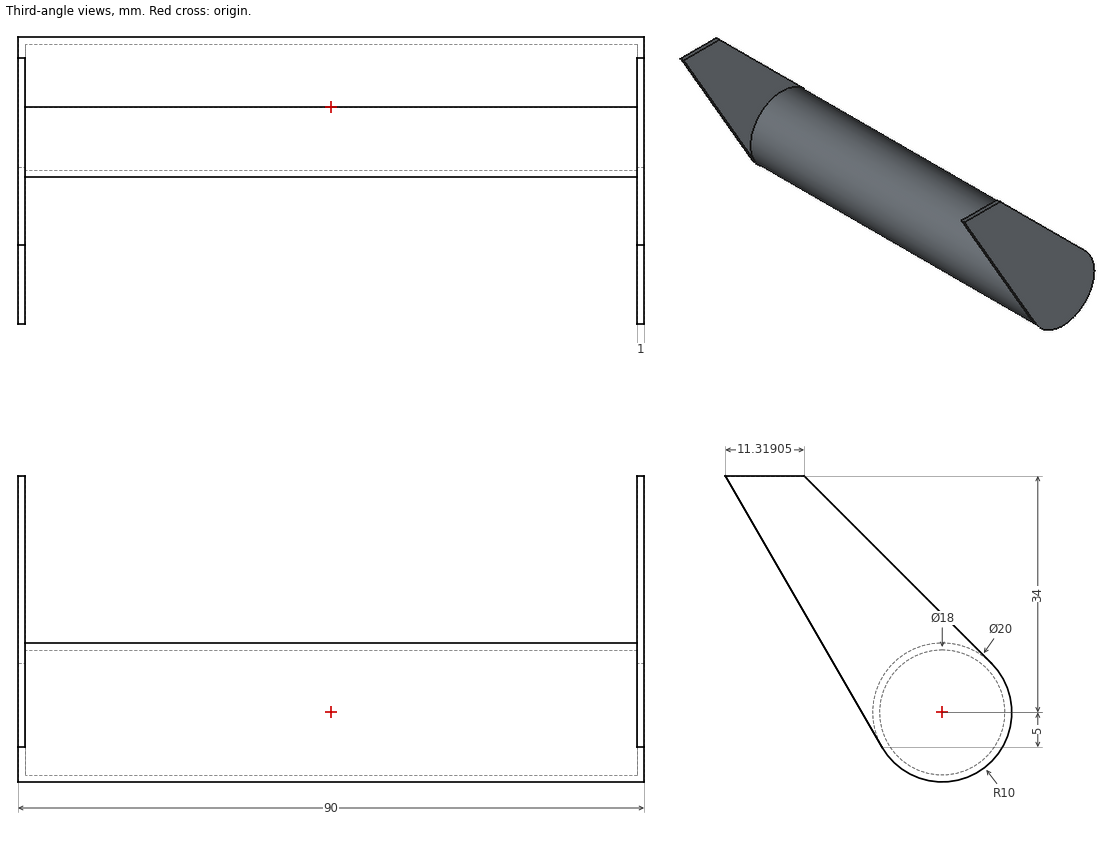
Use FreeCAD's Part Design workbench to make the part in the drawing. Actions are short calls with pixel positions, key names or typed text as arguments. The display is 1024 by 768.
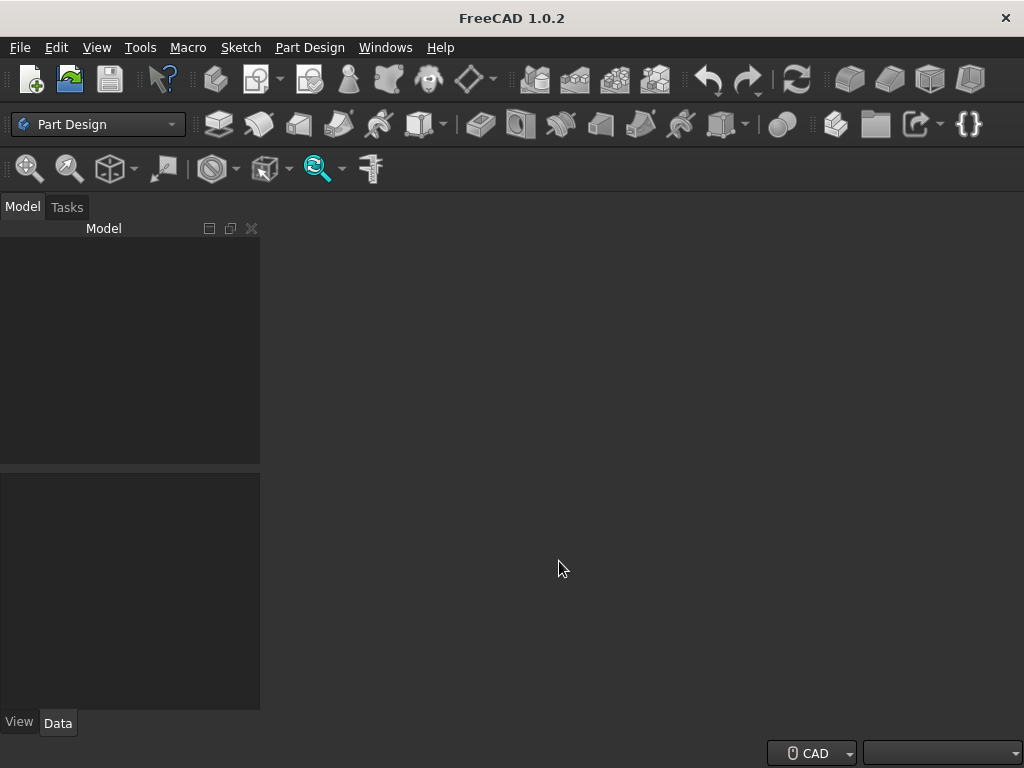
click(30, 80)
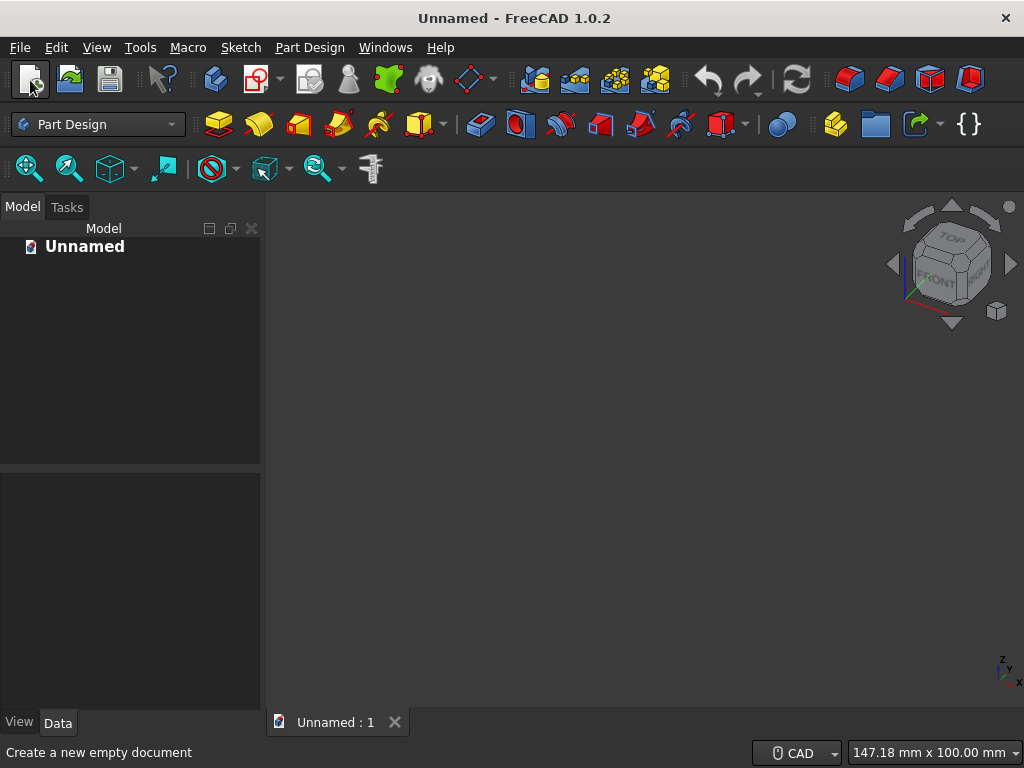
click(256, 80)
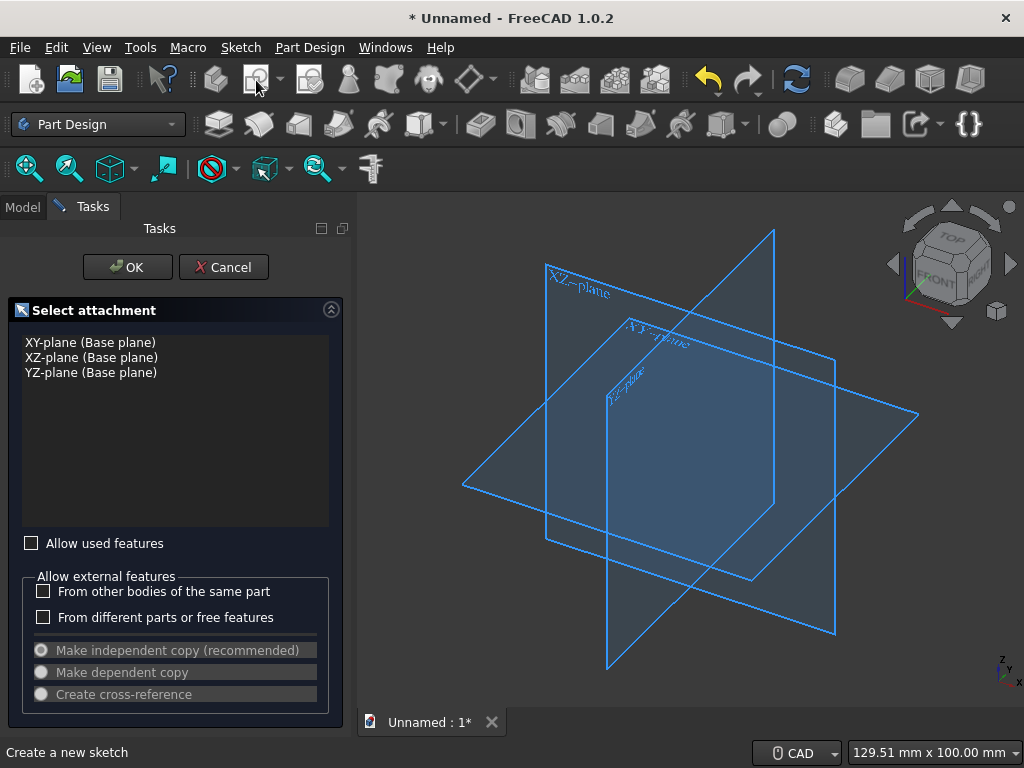
click(82, 372)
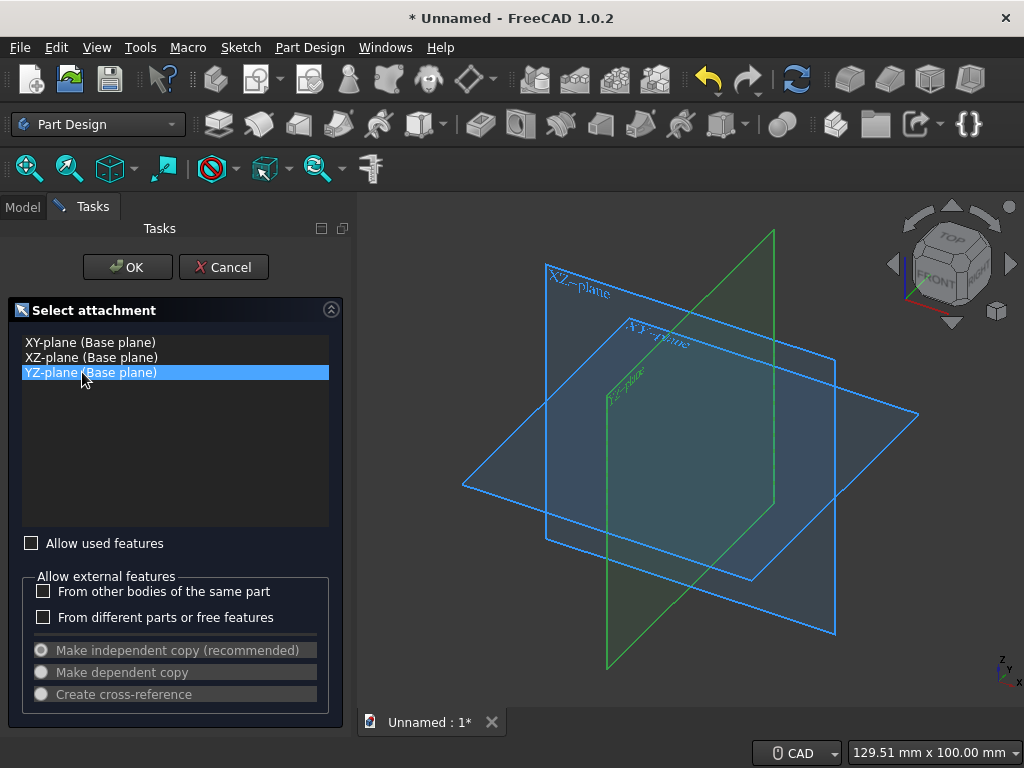
click(128, 267)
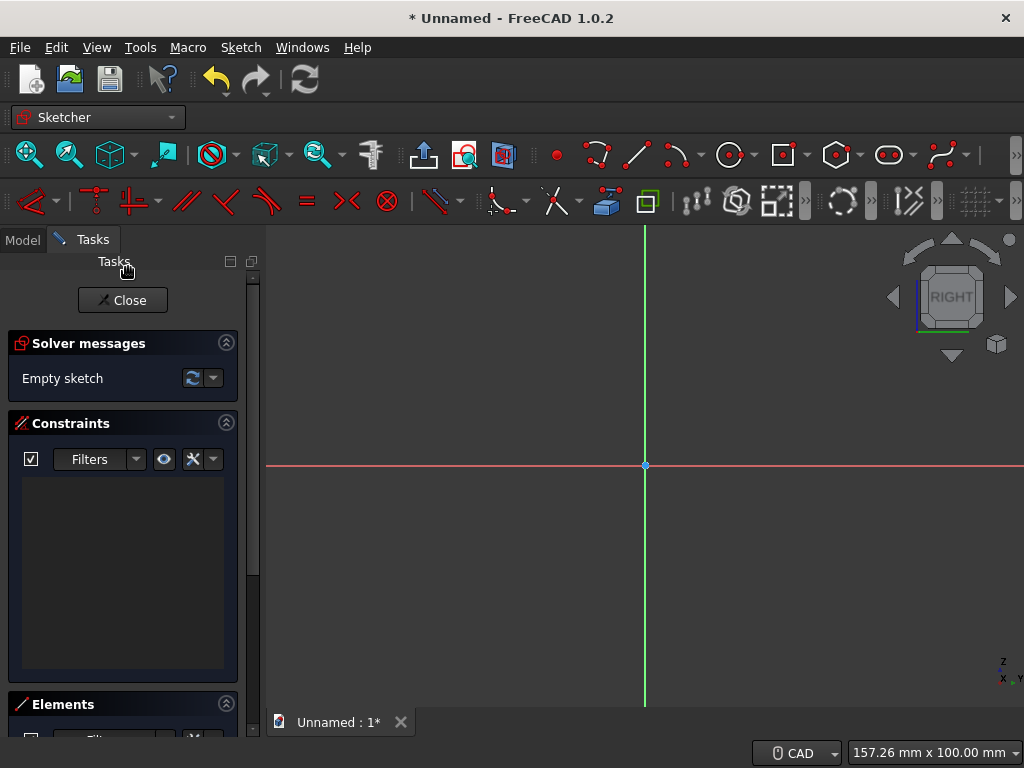
scroll(675, 466, up, 6)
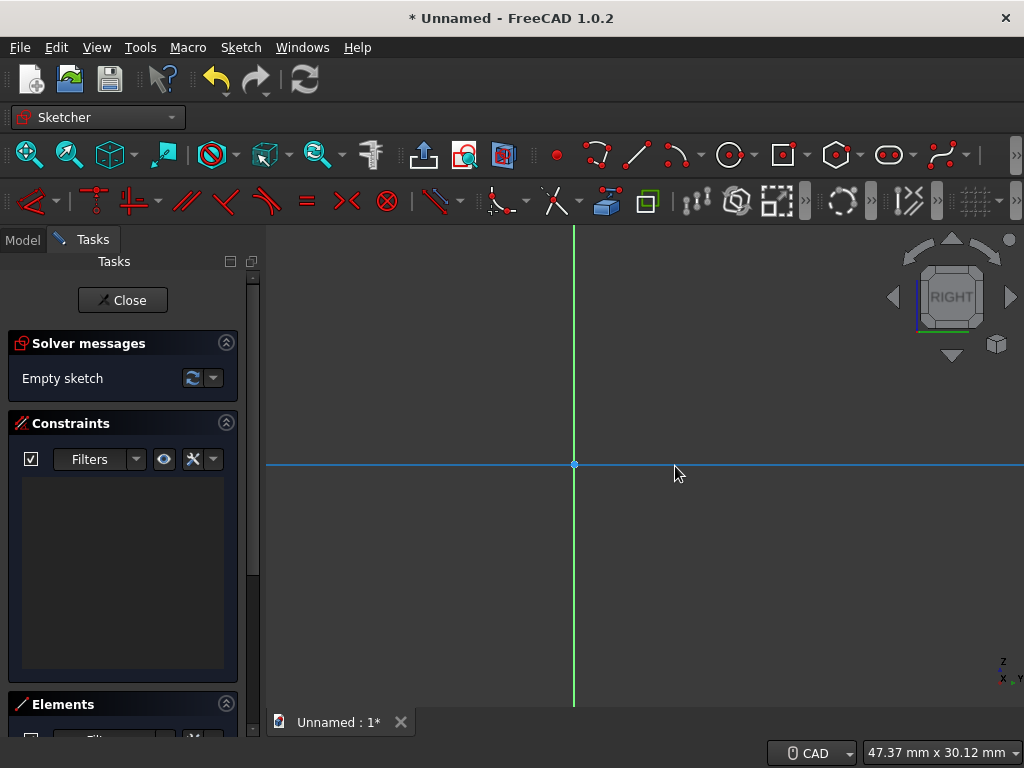
click(730, 156)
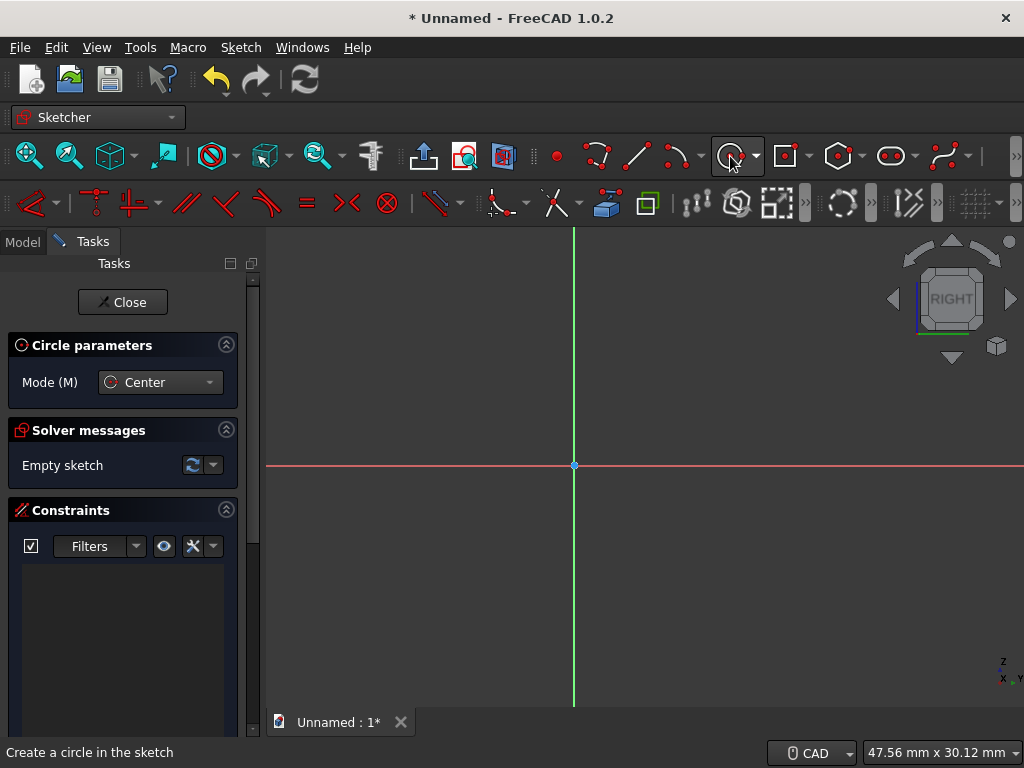
click(574, 466)
click(687, 353)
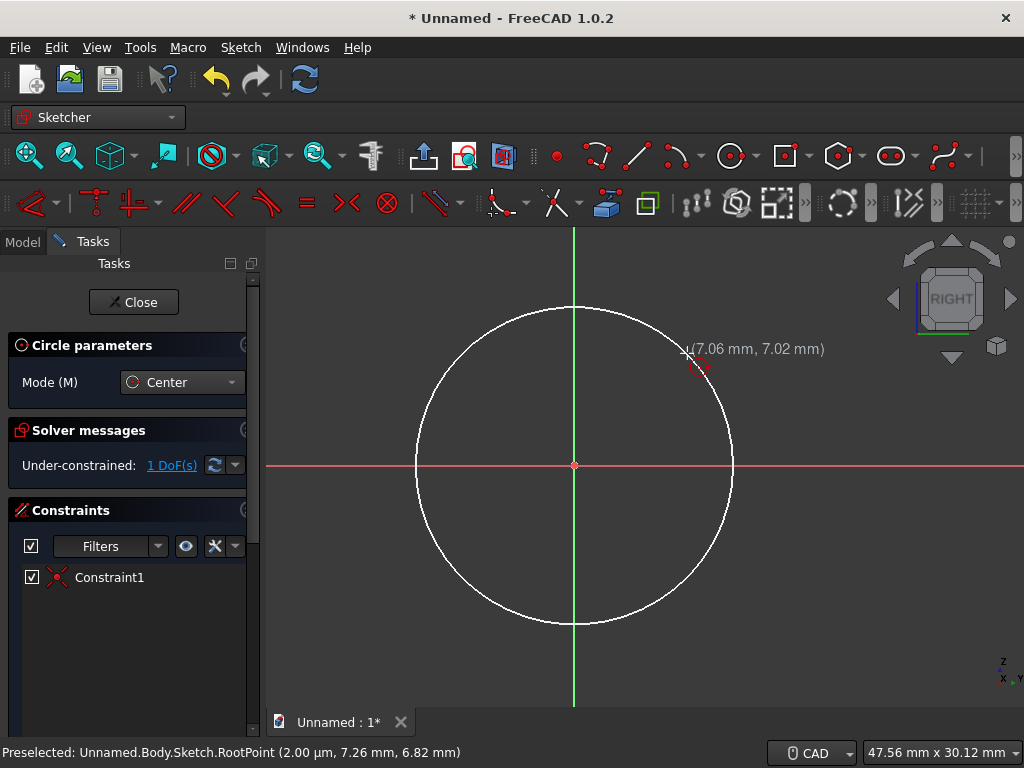
click(574, 466)
click(676, 364)
key(Escape)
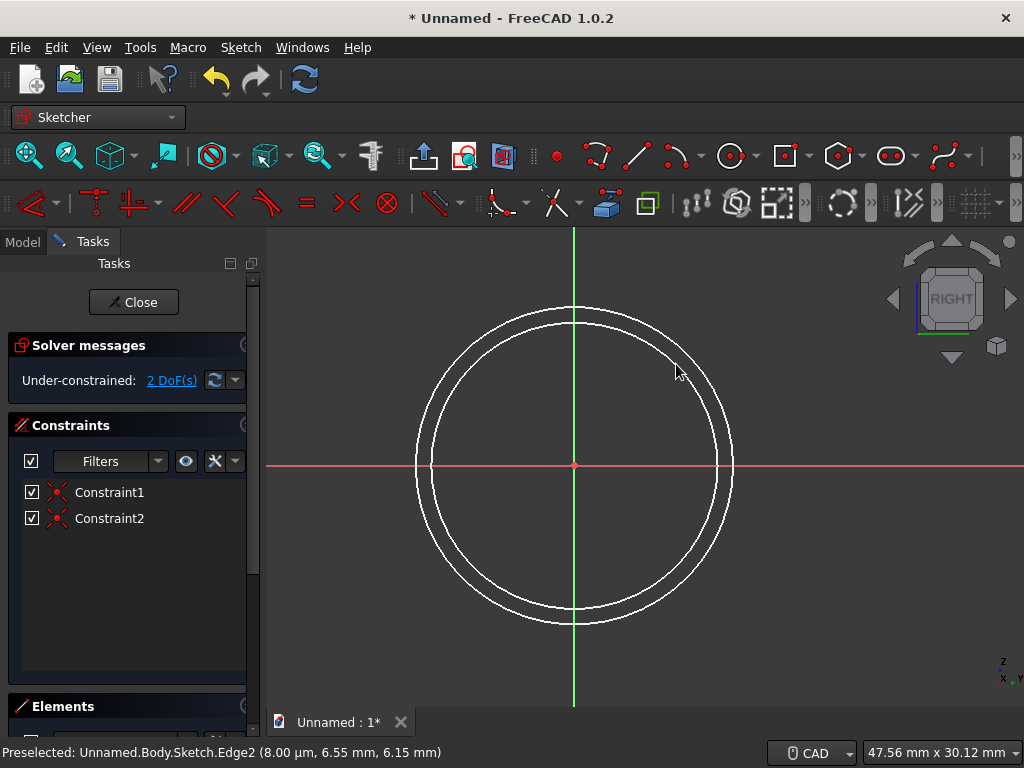
click(32, 204)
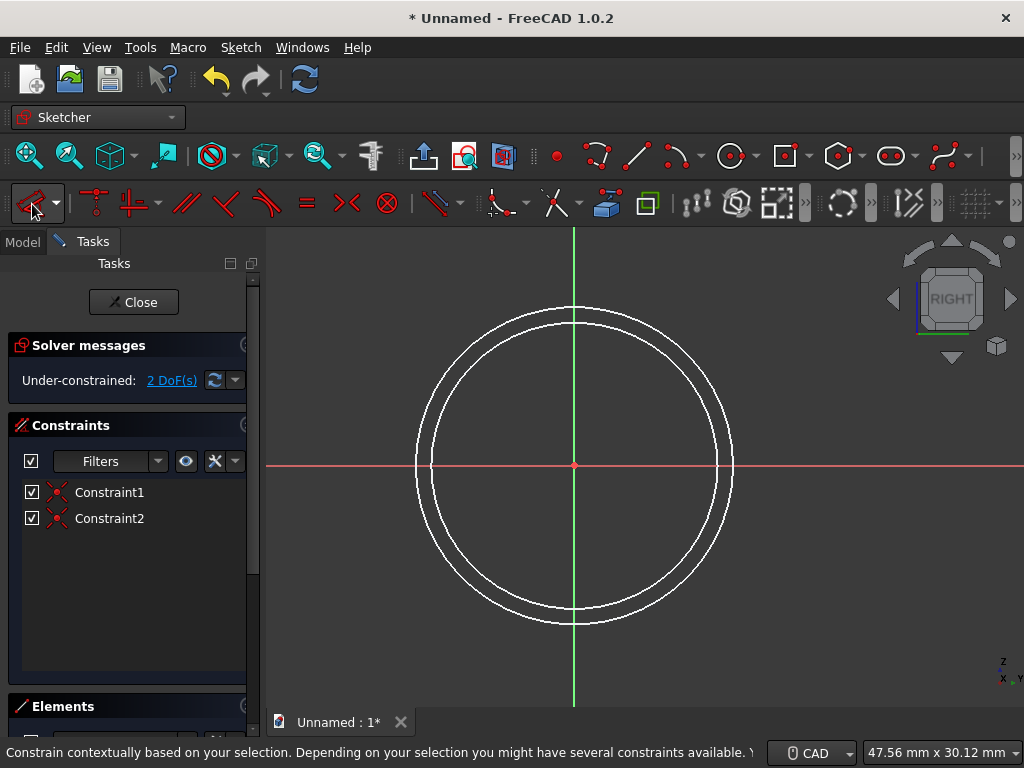
click(686, 353)
click(708, 330)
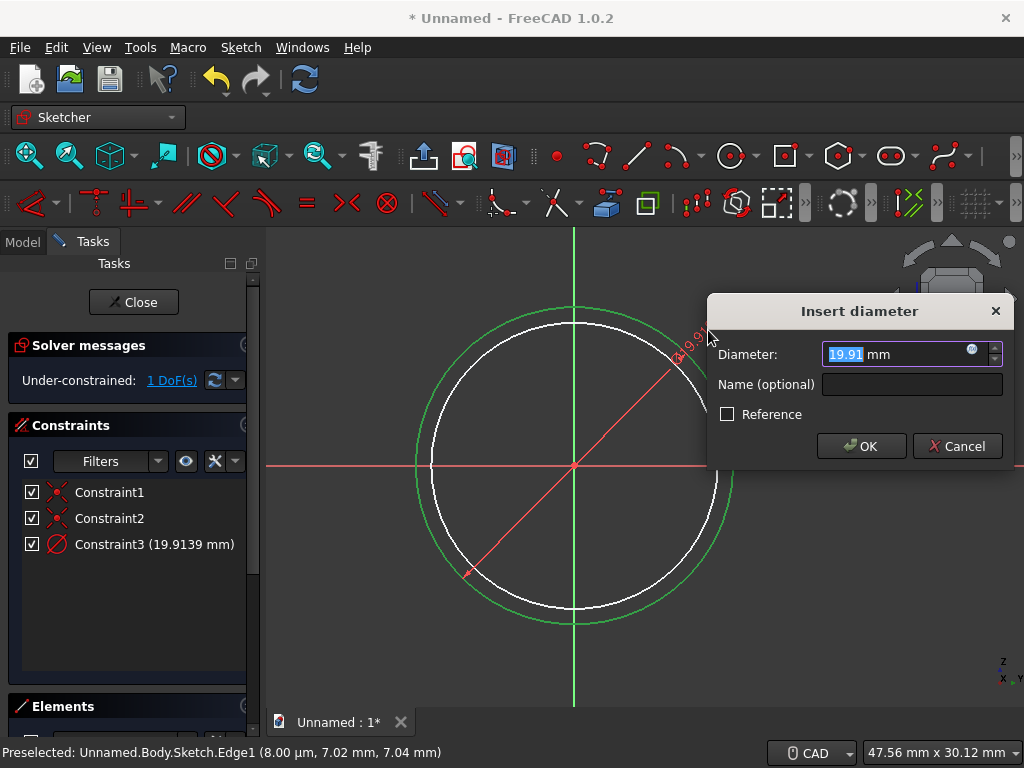
text(20)
key(Return)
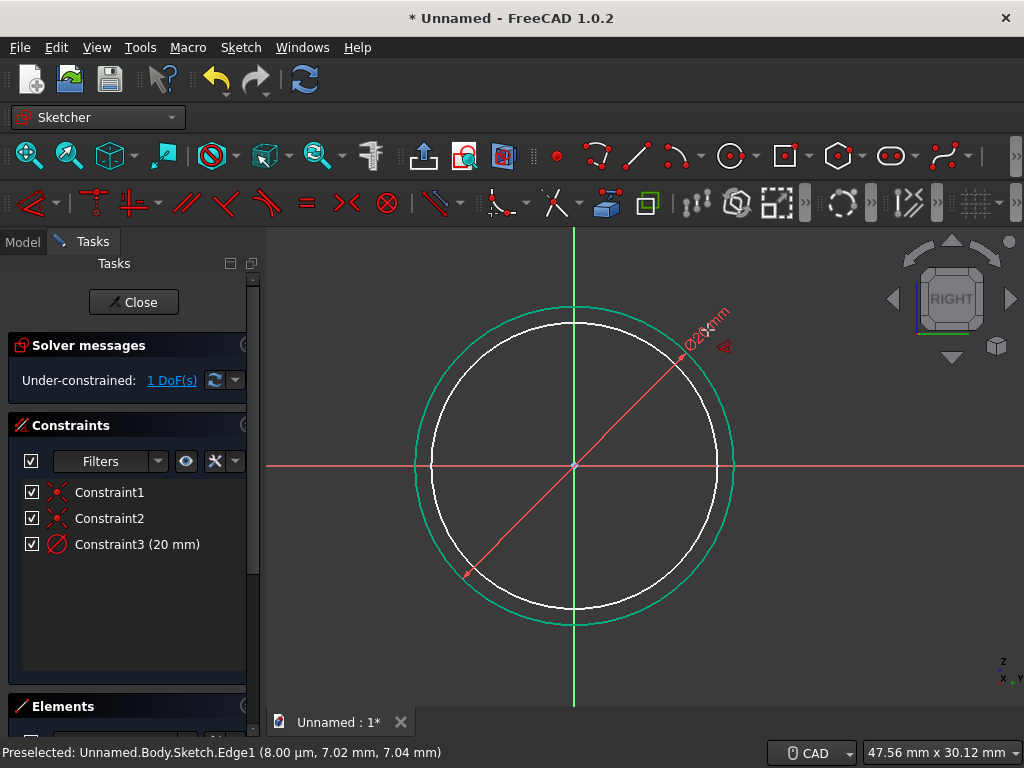
click(675, 364)
click(742, 415)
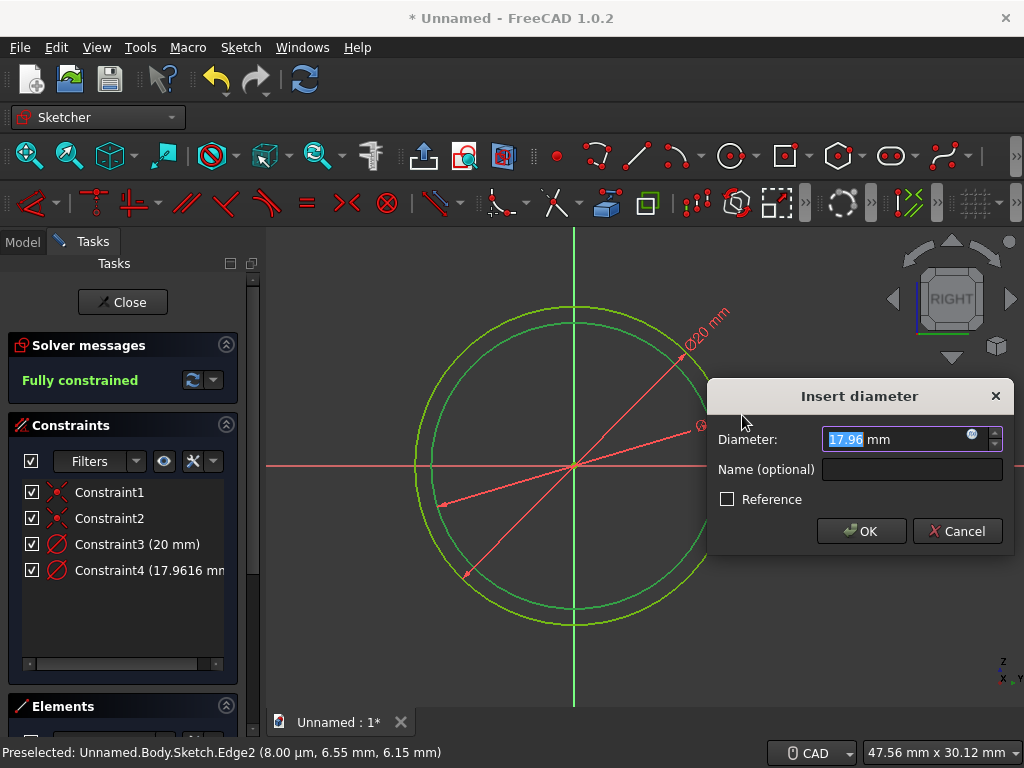
text(18)
key(Return)
key(Escape)